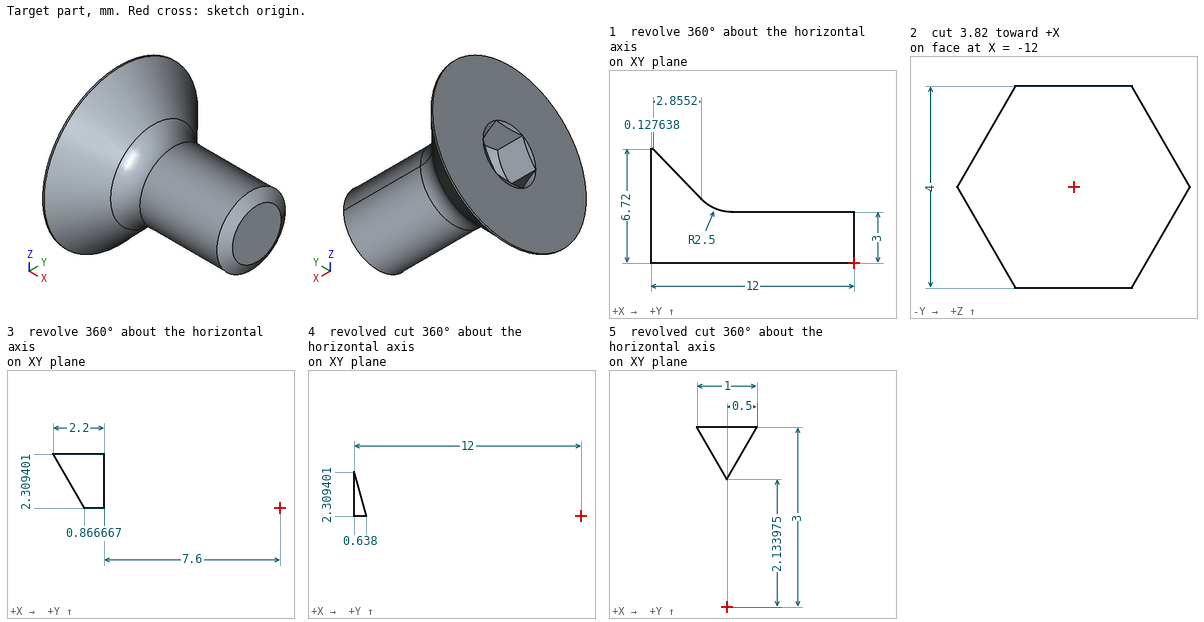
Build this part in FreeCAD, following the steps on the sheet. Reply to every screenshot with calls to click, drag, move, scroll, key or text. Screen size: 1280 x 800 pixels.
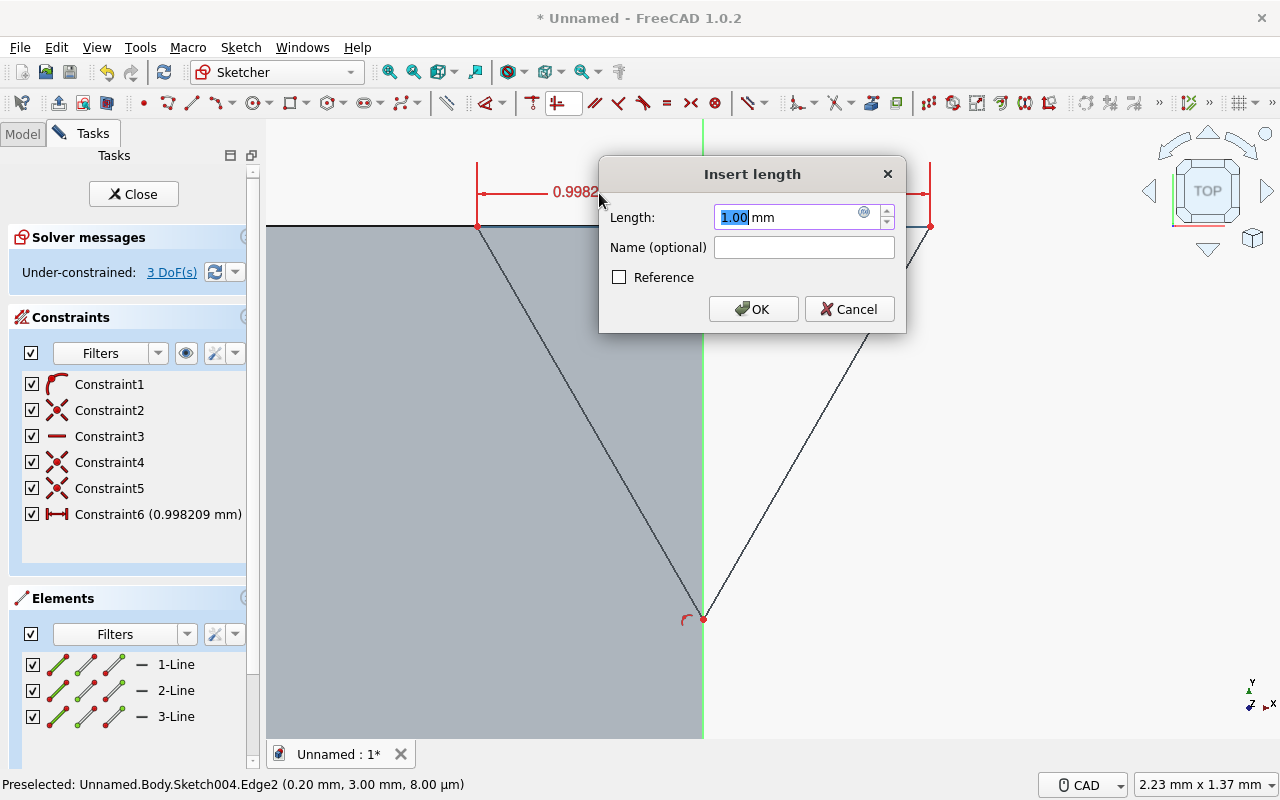
text(1)
key(Return)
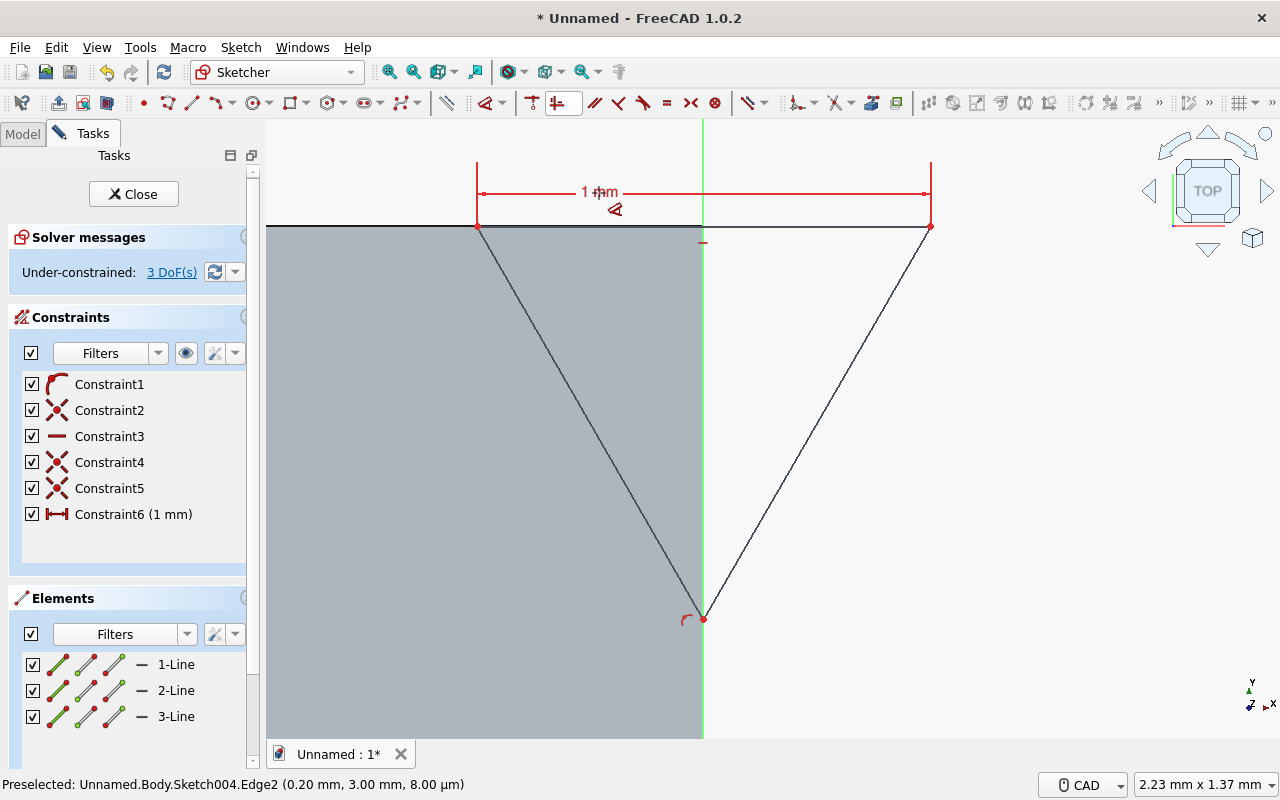
click(931, 227)
click(965, 469)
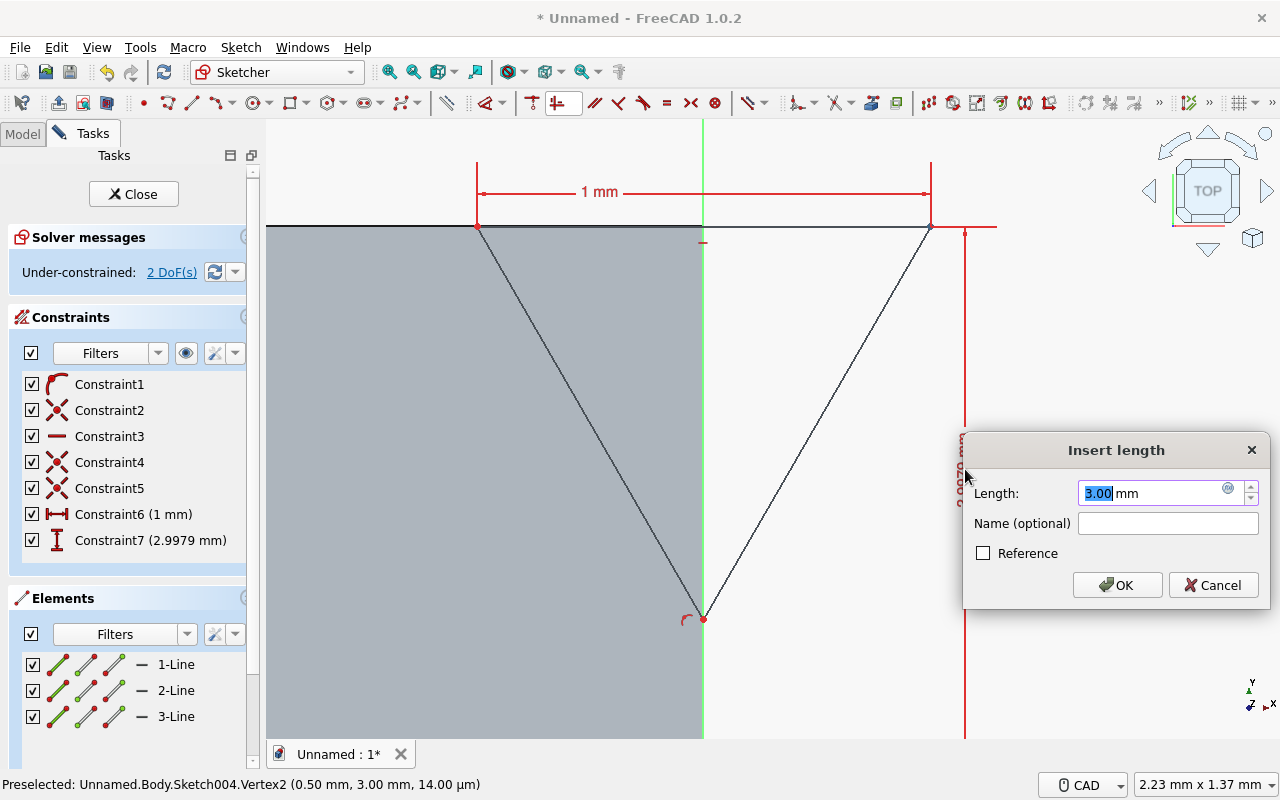
text(3)
key(Return)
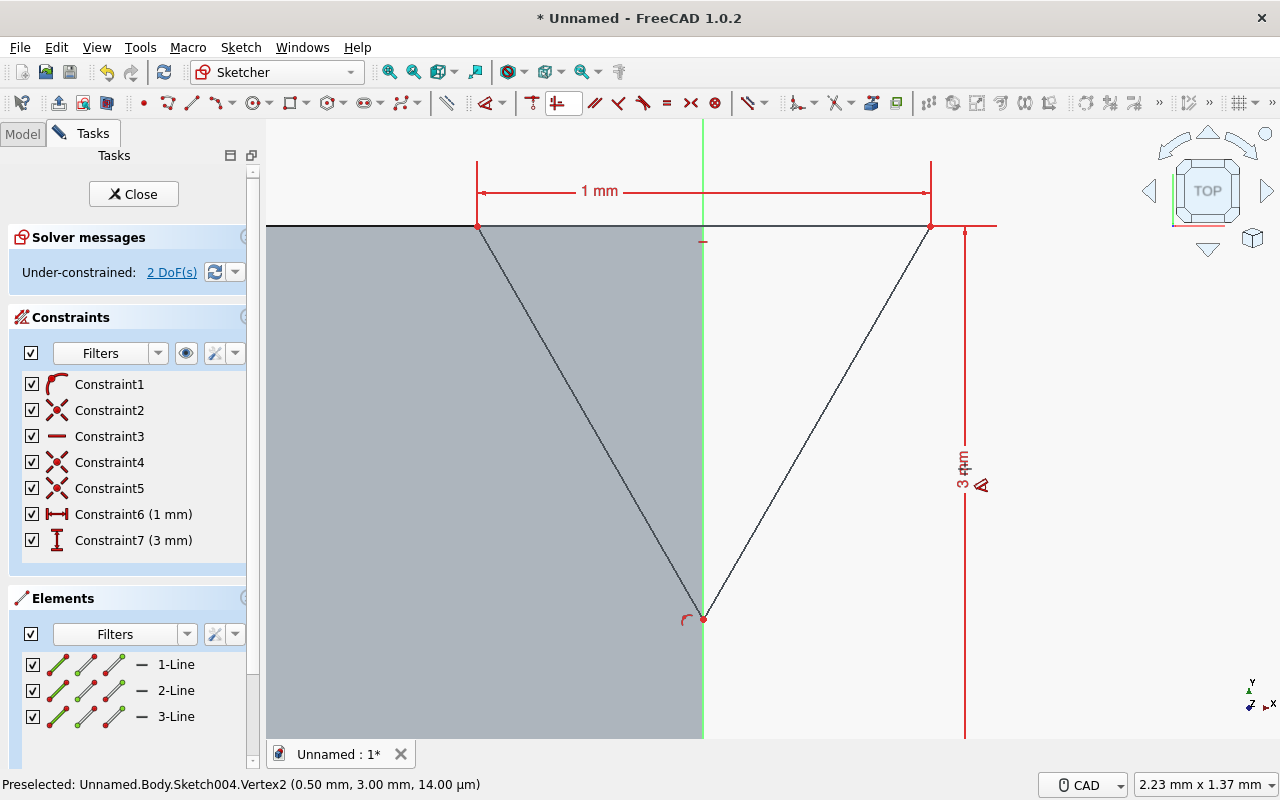
click(931, 226)
click(817, 192)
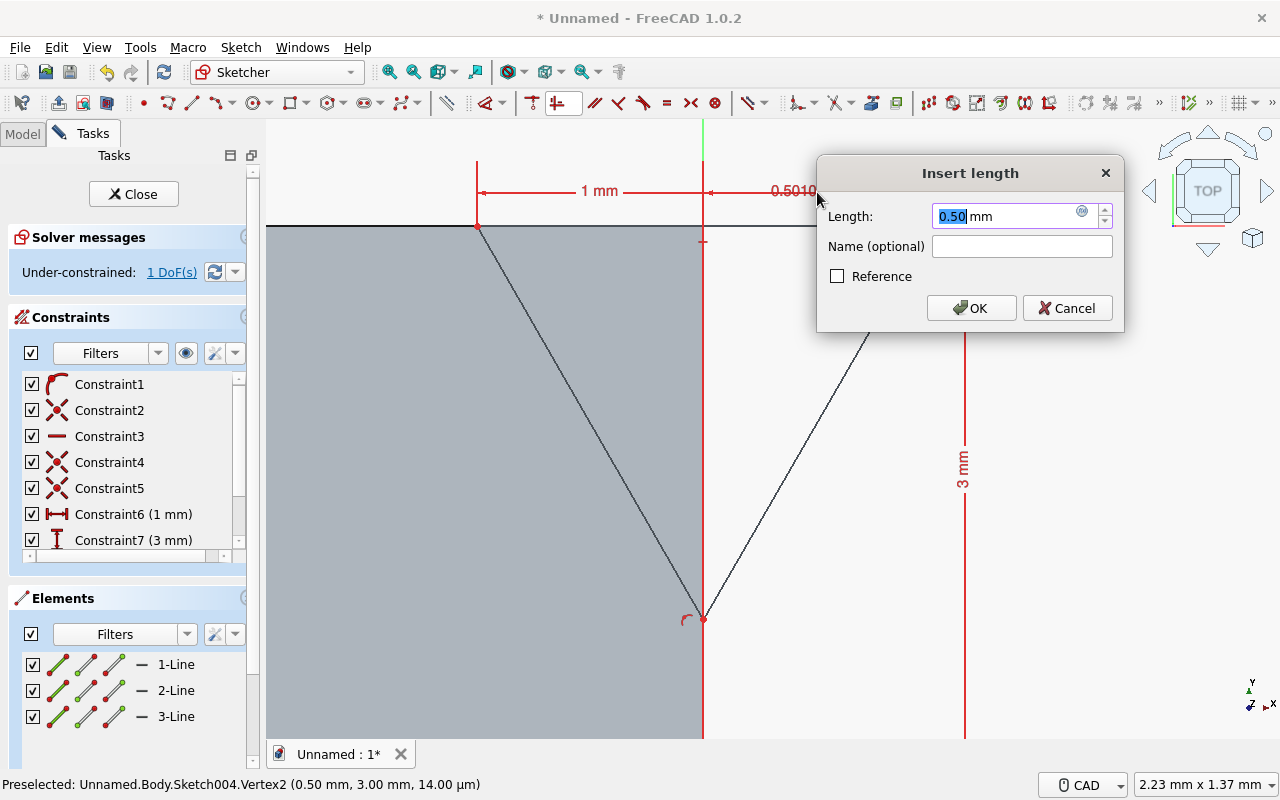
text(0.5)
key(Return)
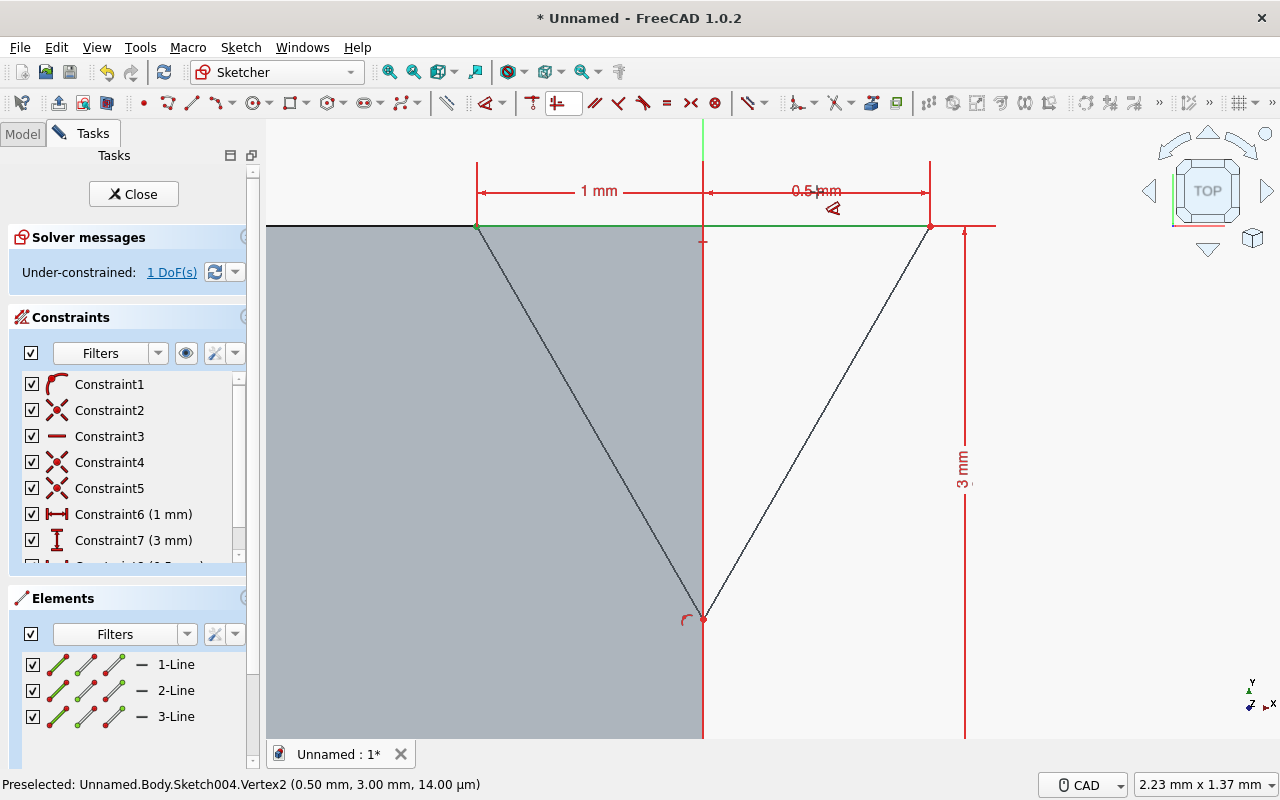
click(703, 620)
click(737, 665)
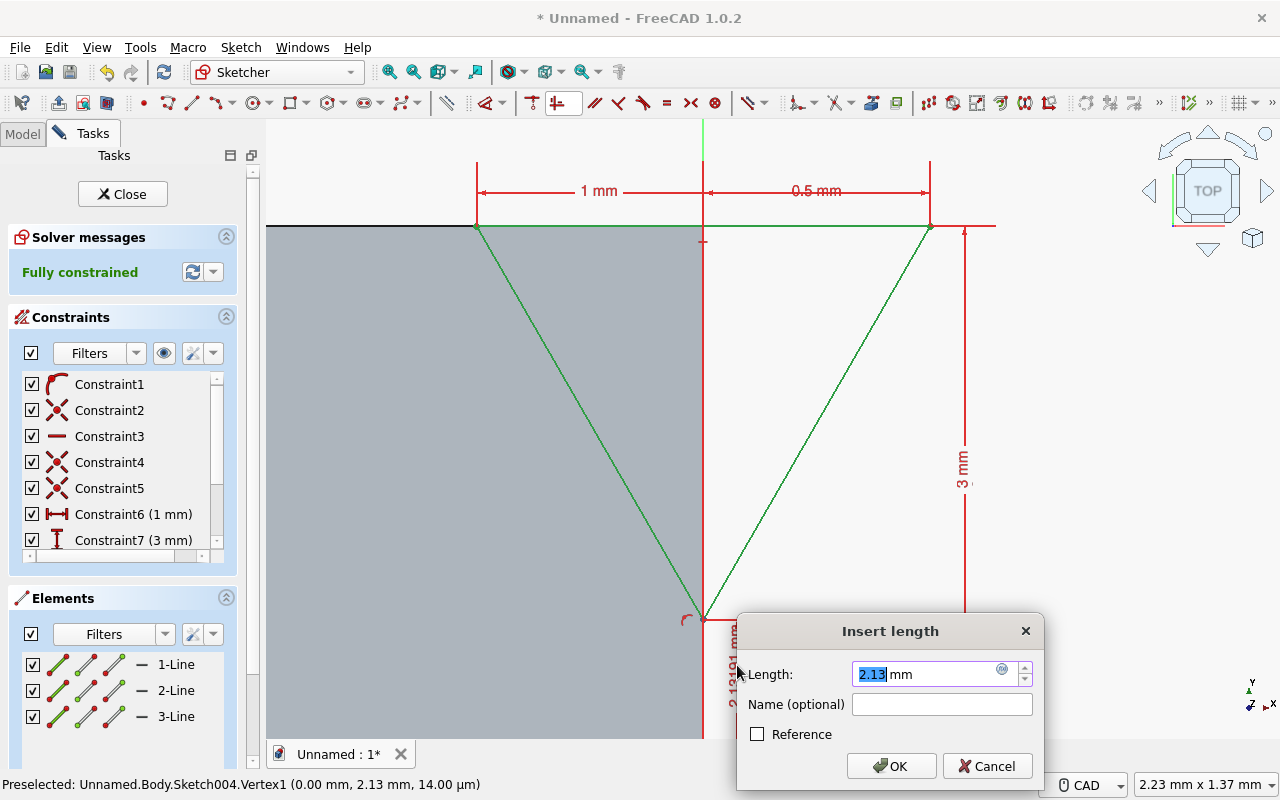
text(2.133975)
key(Return)
key(Escape)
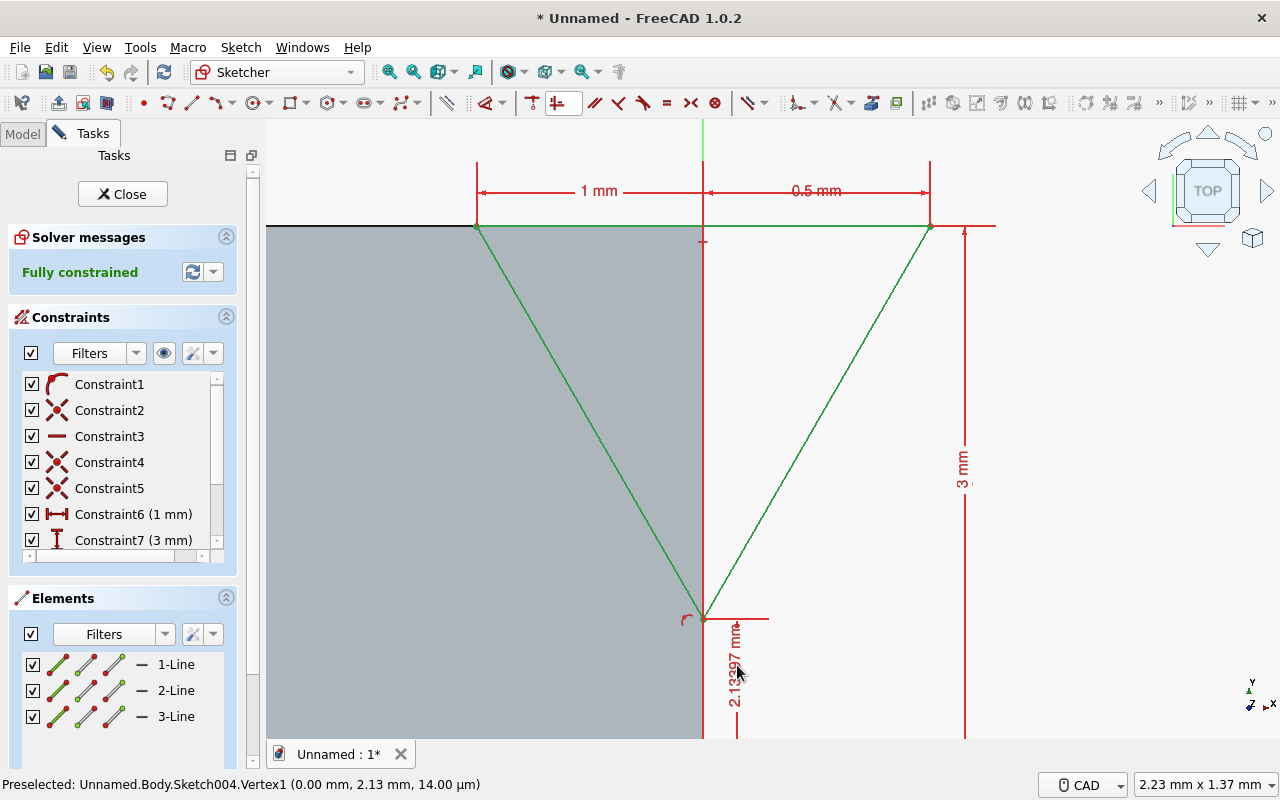
click(123, 194)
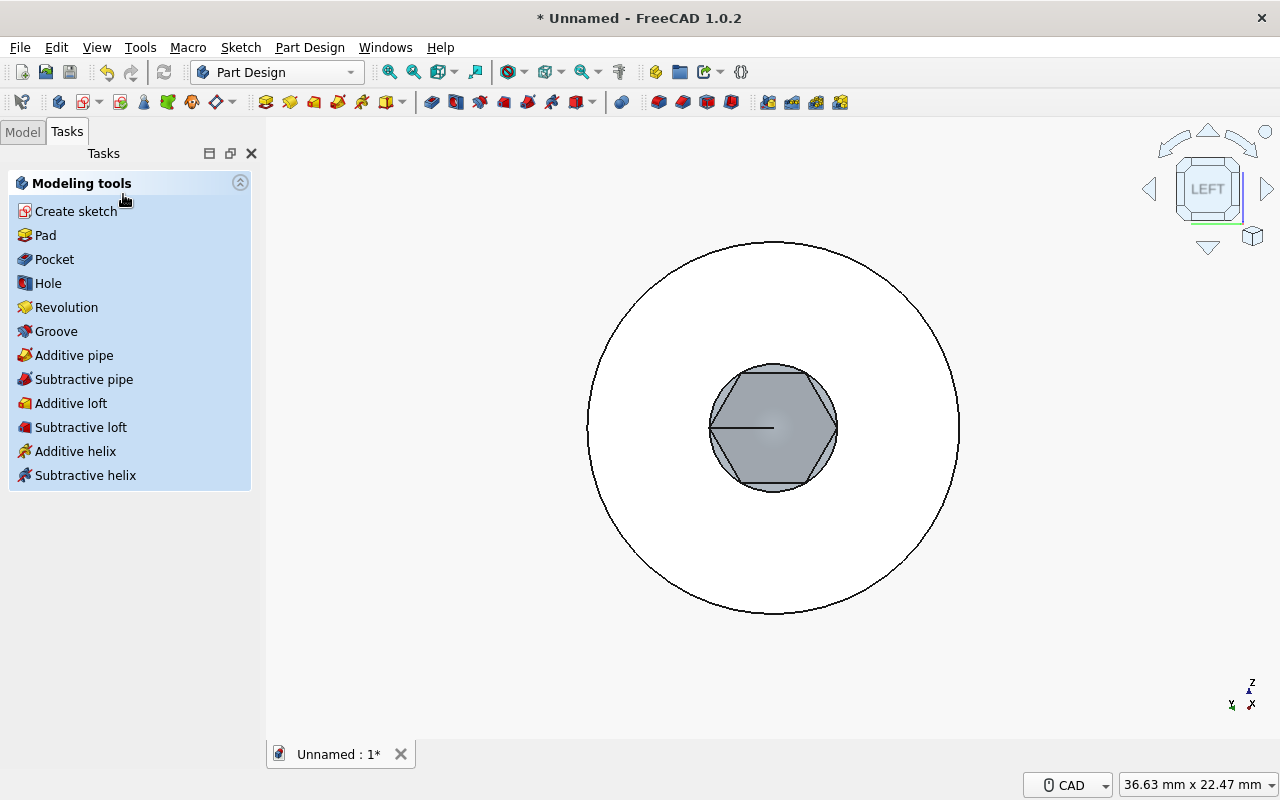
click(480, 102)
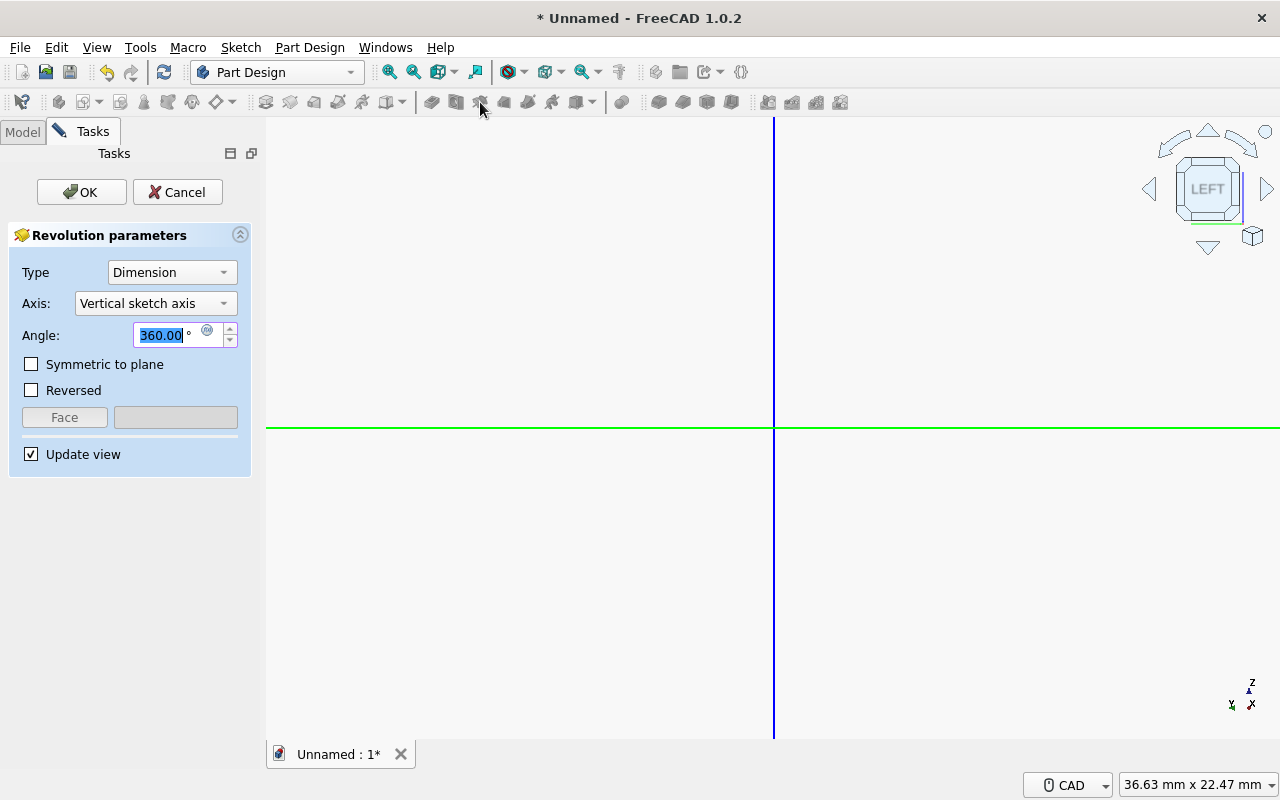
click(156, 304)